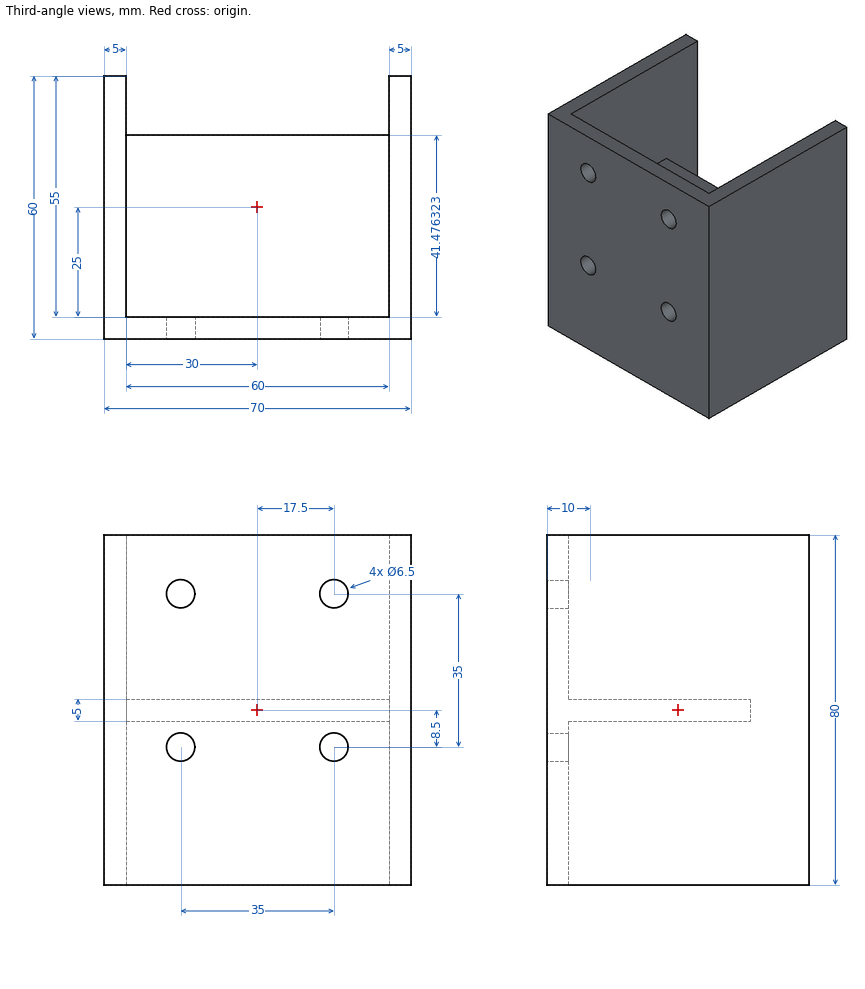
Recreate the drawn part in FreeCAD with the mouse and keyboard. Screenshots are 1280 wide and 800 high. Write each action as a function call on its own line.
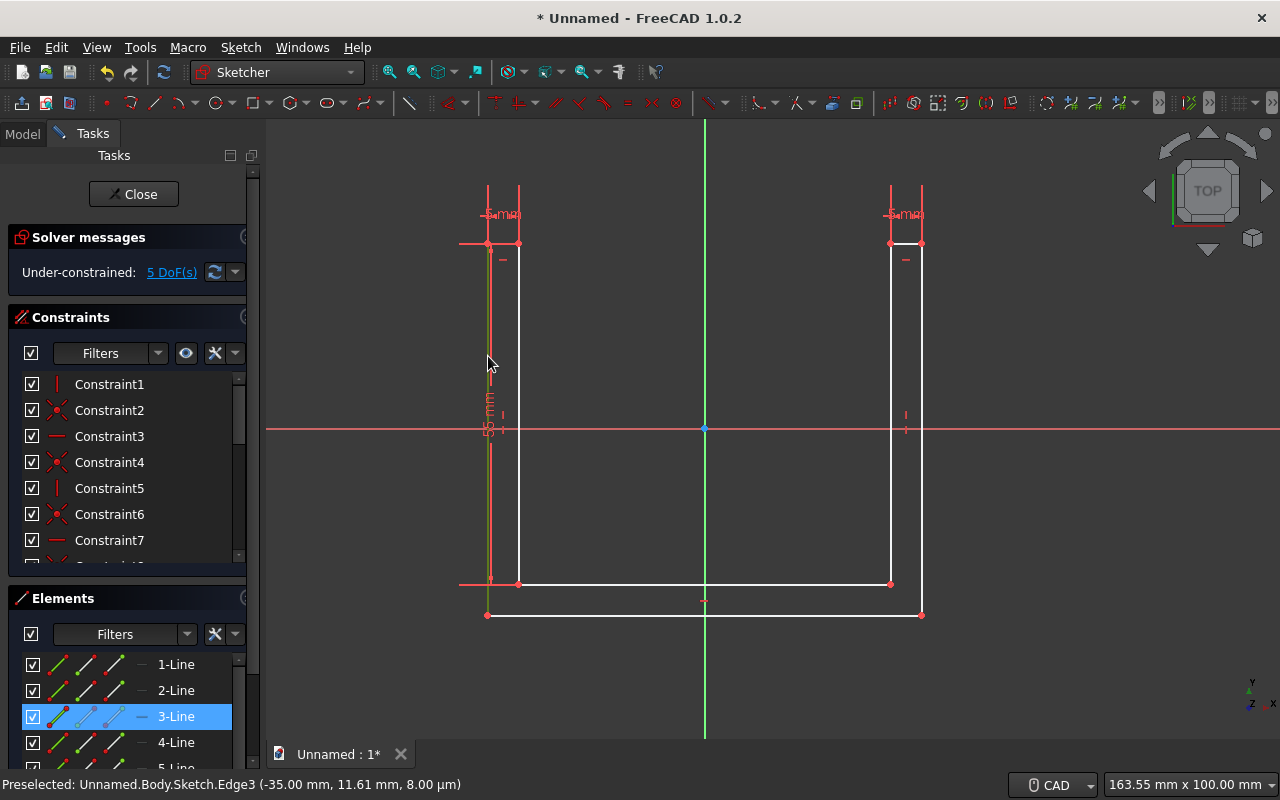
key(i)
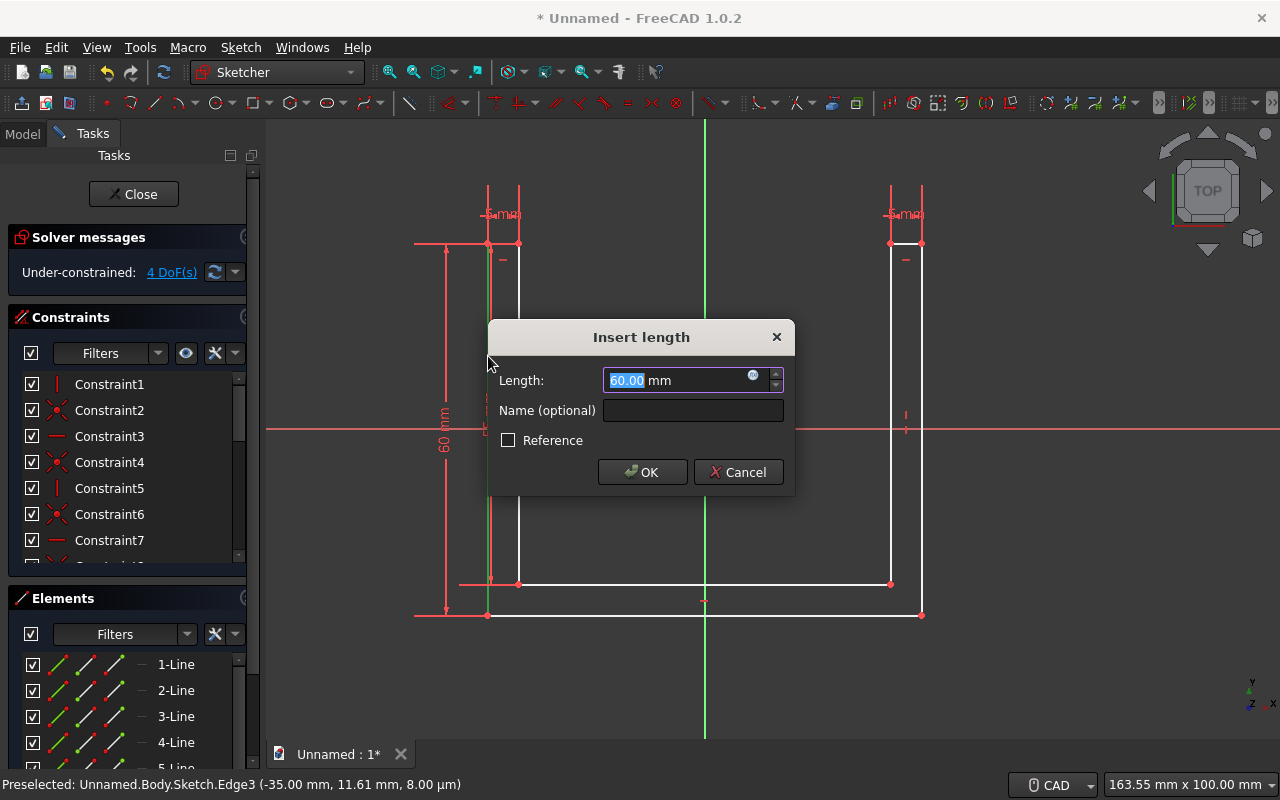
text(60)
key(Return)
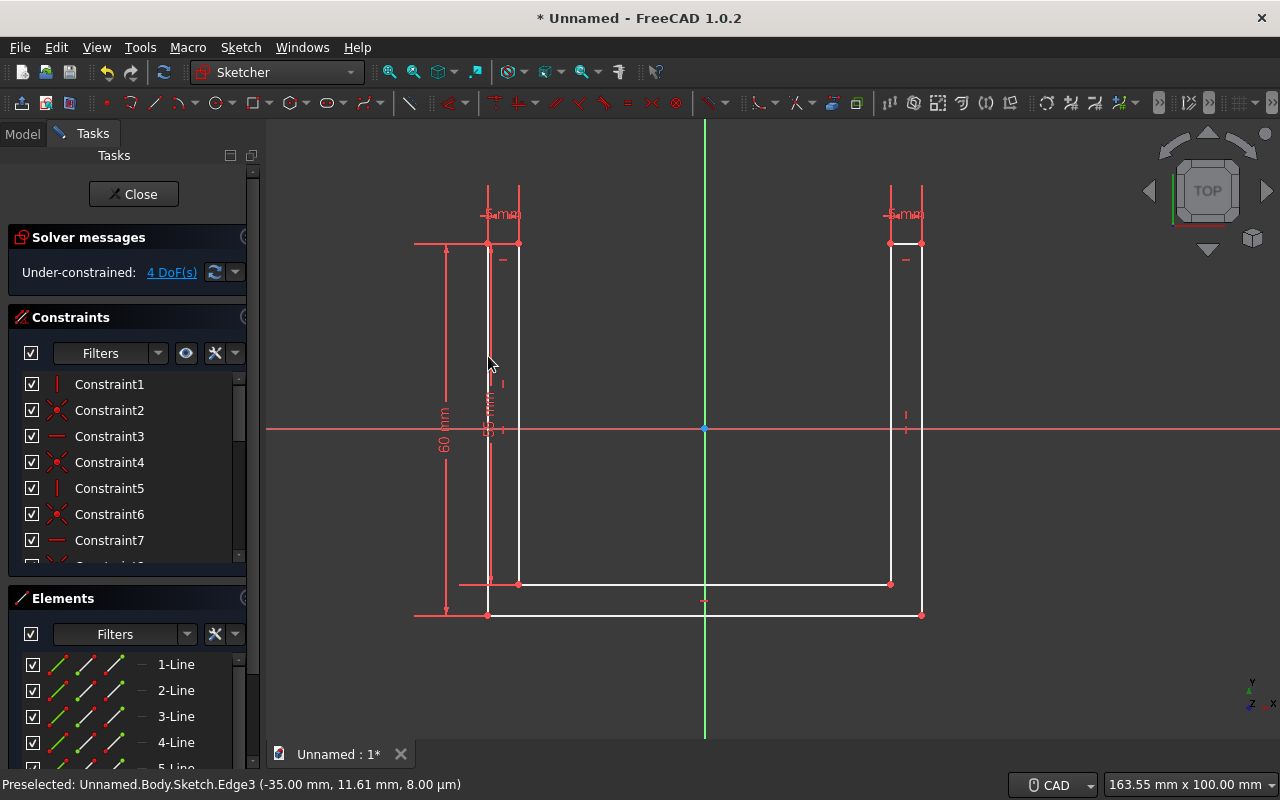
click(618, 616)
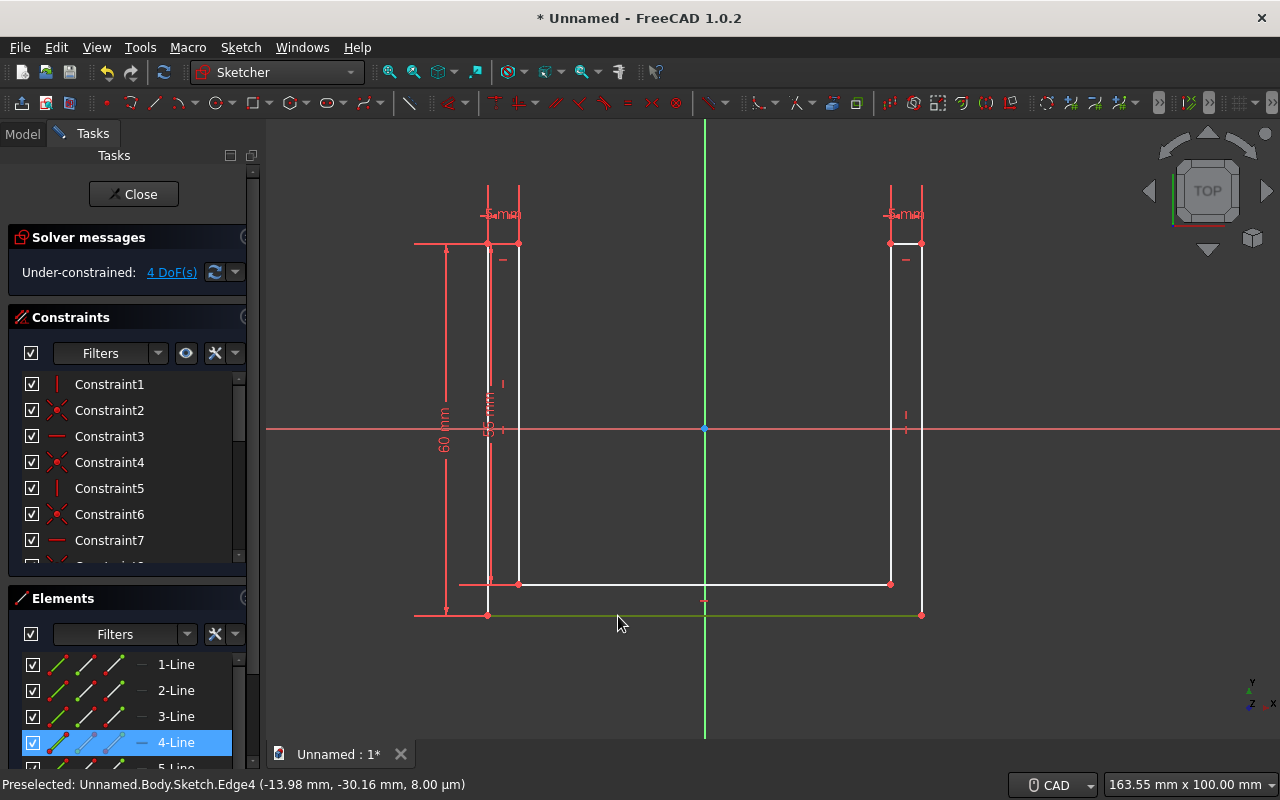
key(l)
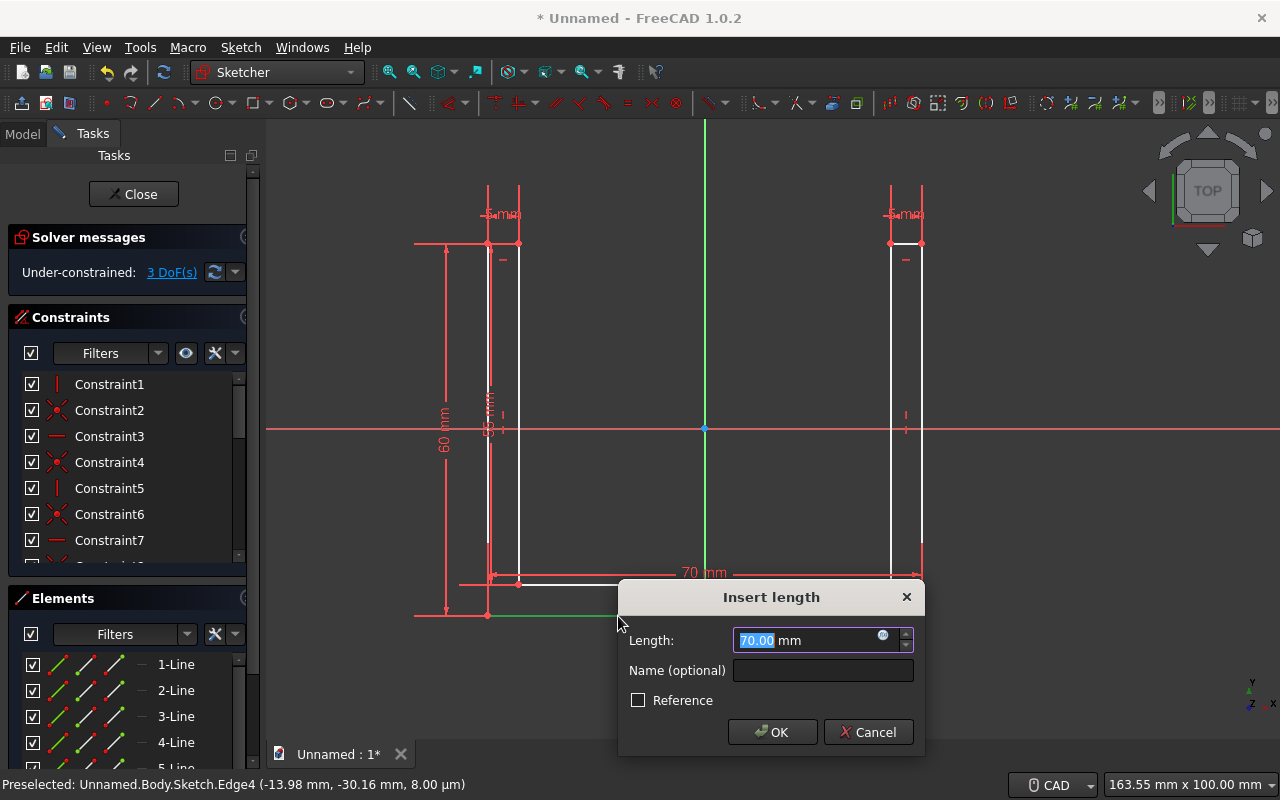
text(70)
key(Return)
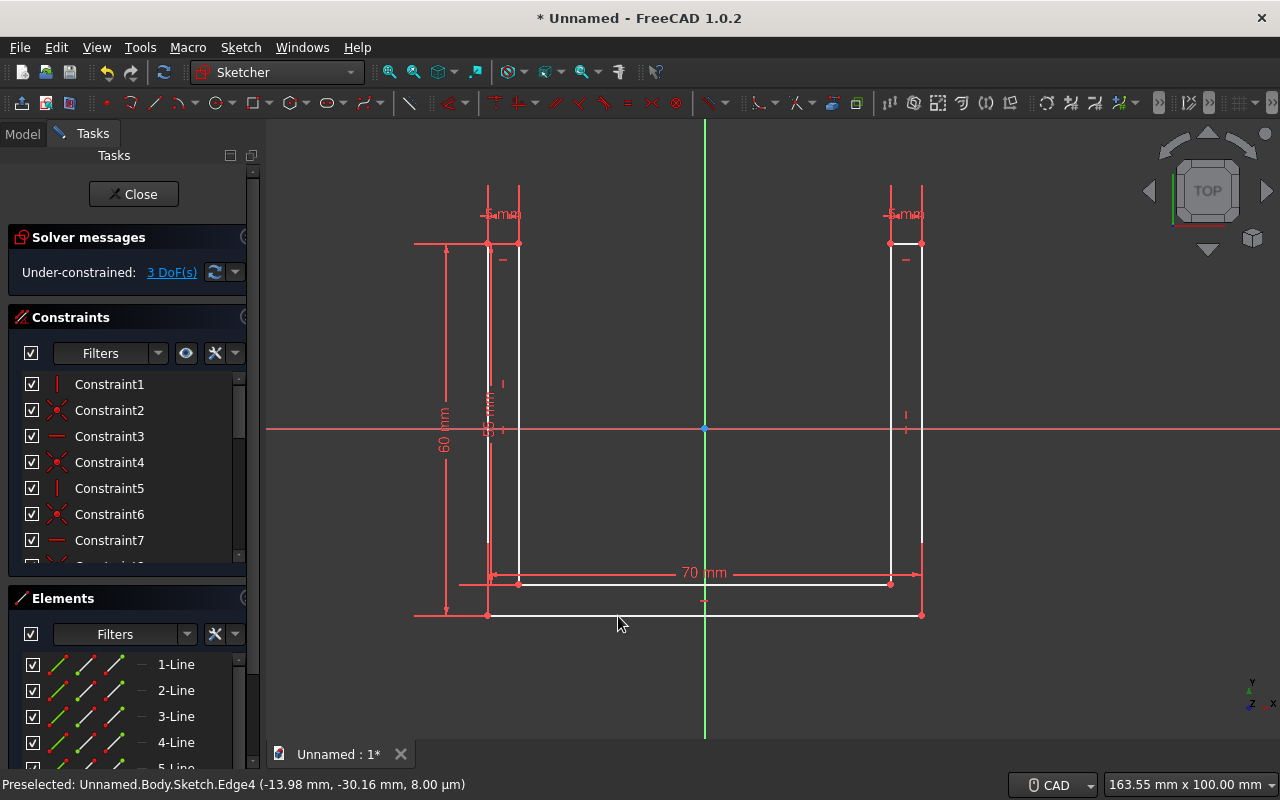
click(922, 504)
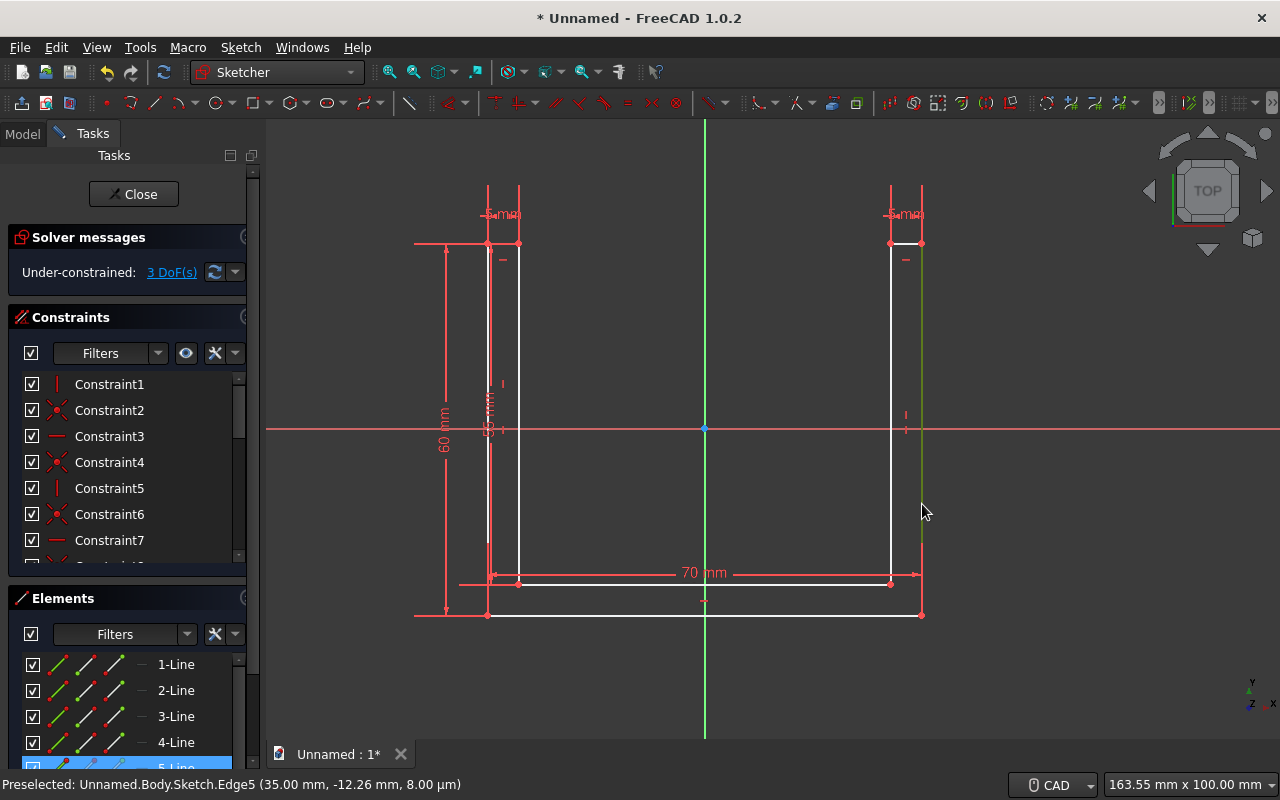
key(i)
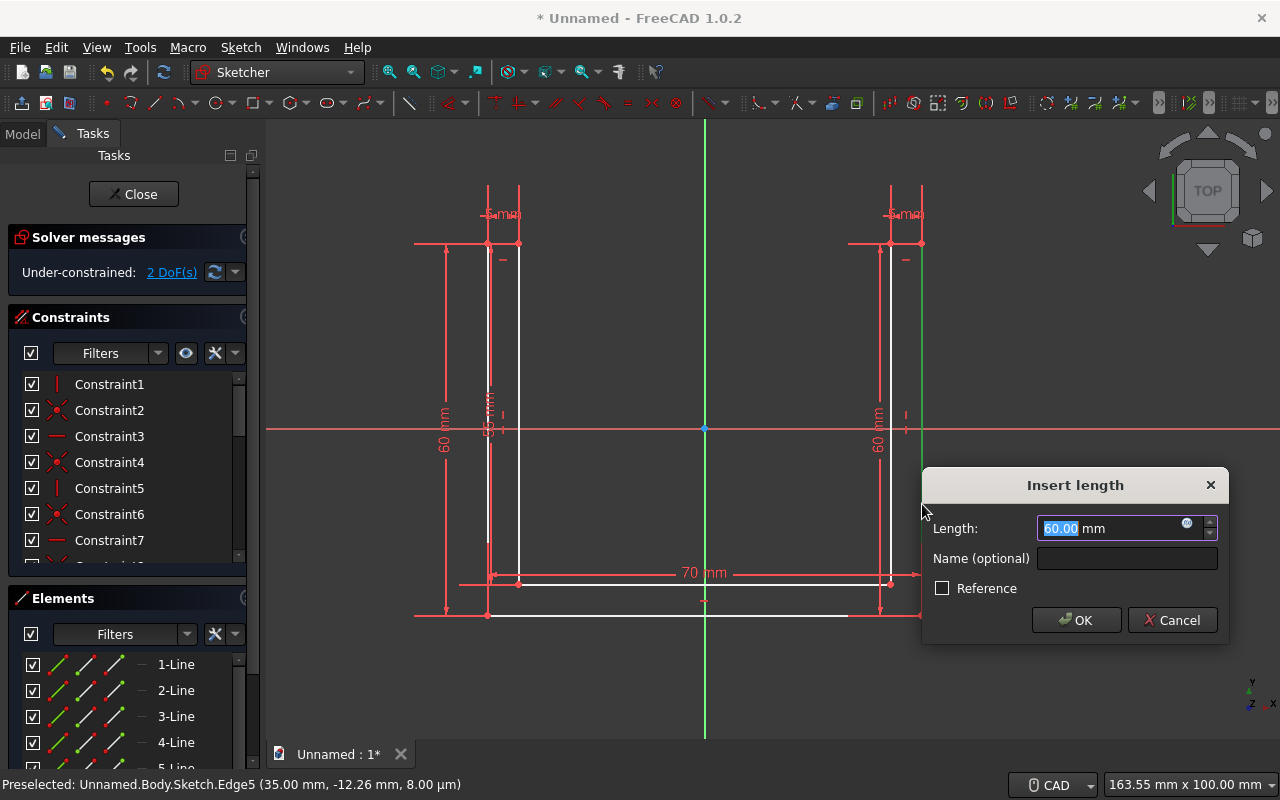
text(60)
key(Return)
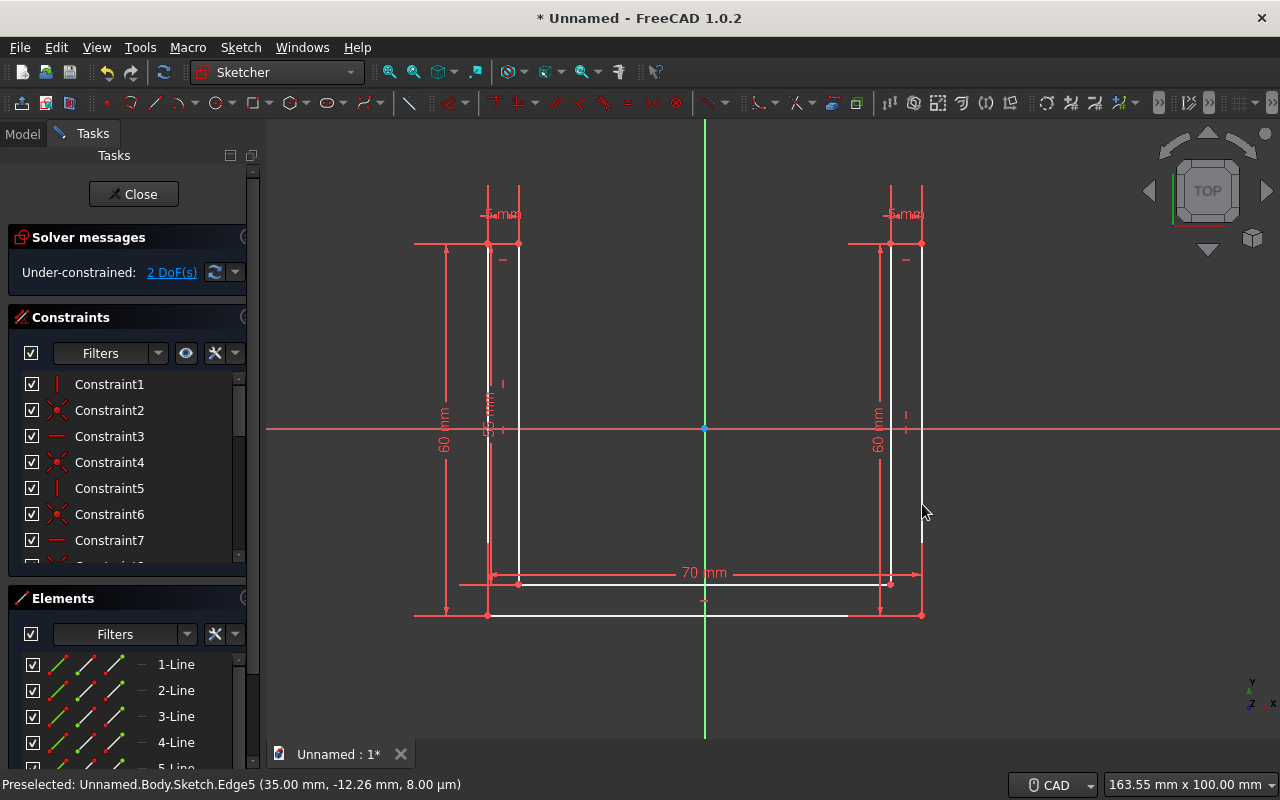
click(519, 585)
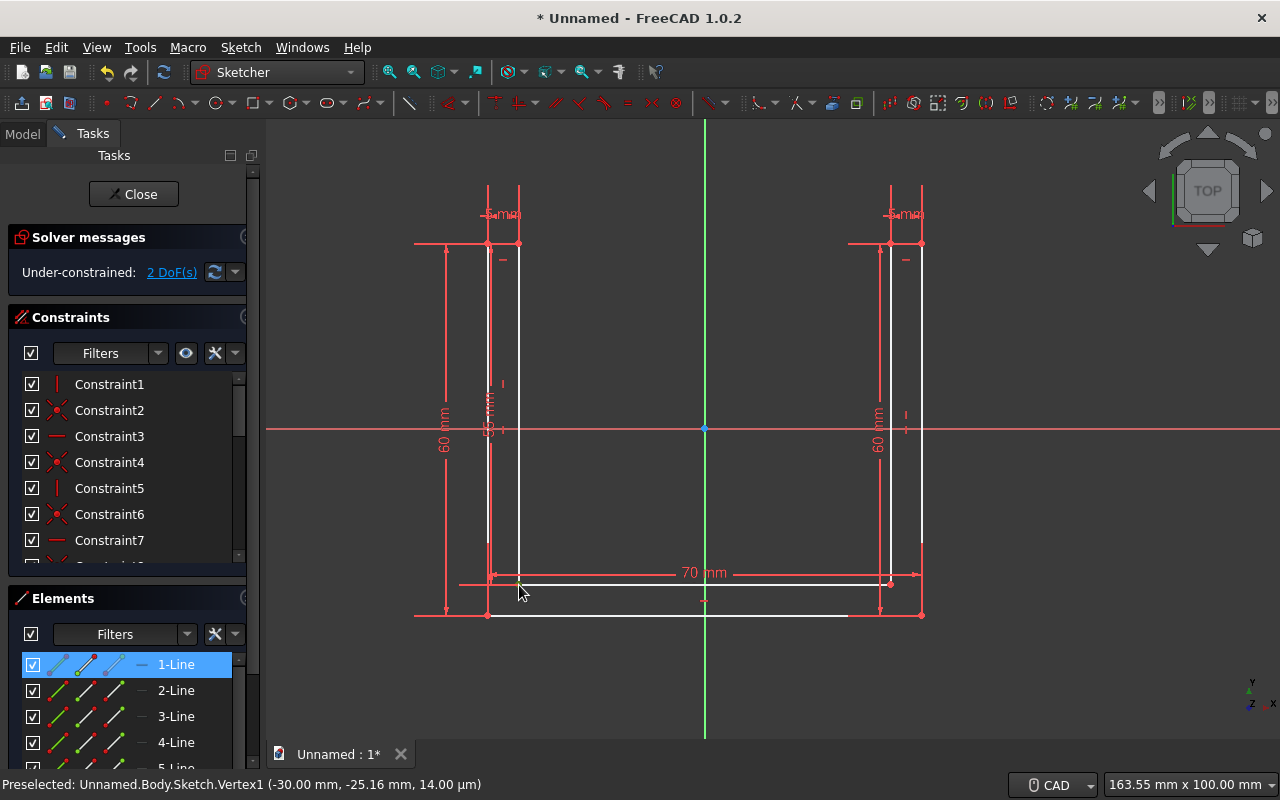
key(l)